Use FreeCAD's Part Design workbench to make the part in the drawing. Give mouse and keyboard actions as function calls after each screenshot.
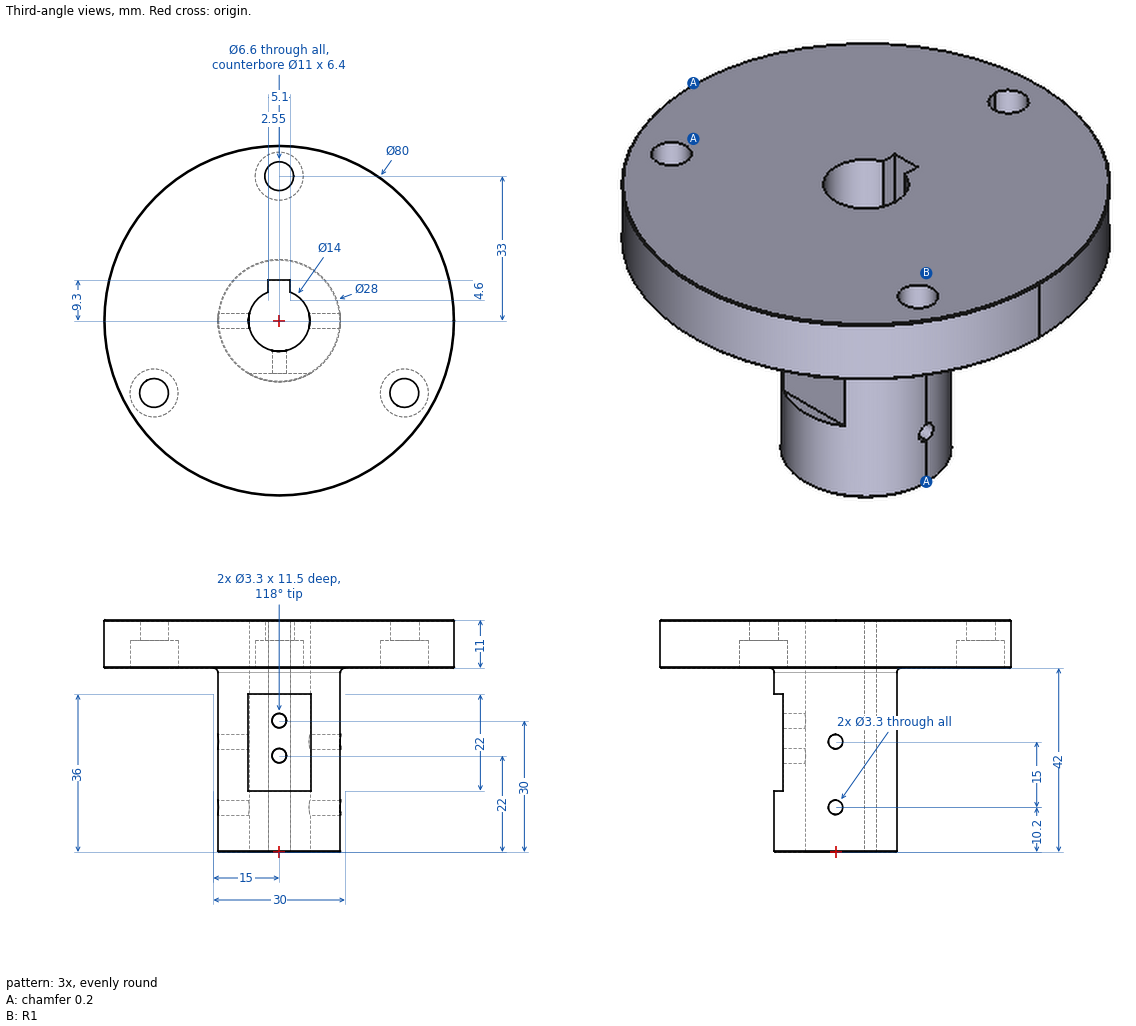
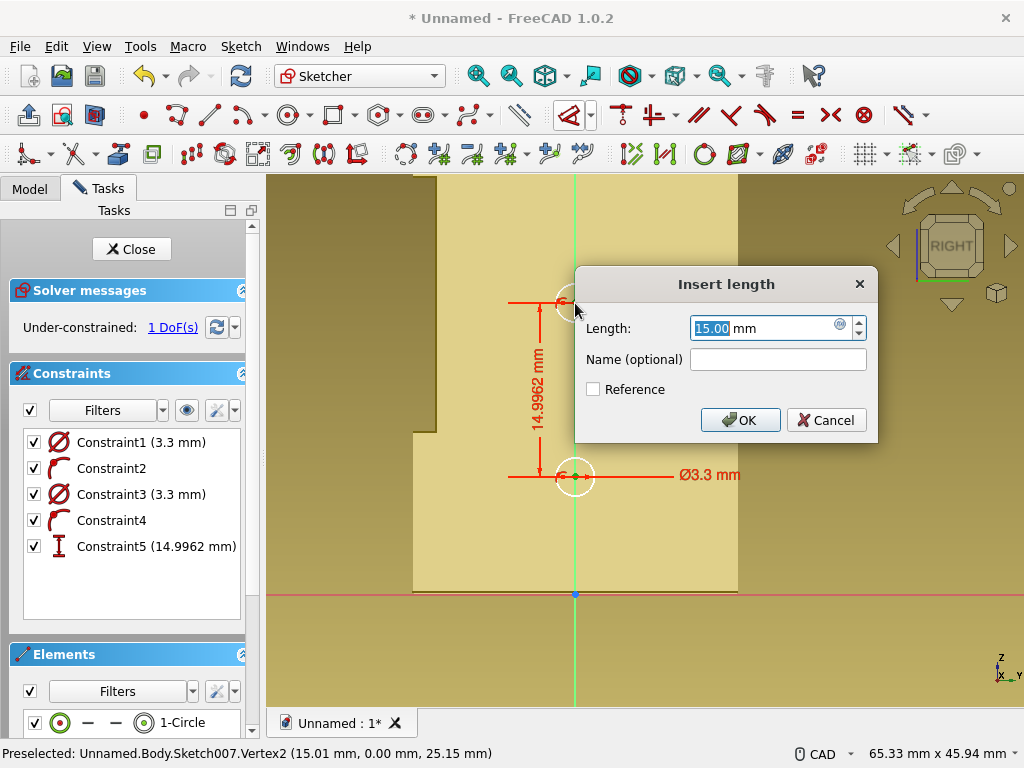
text(15)
key(Return)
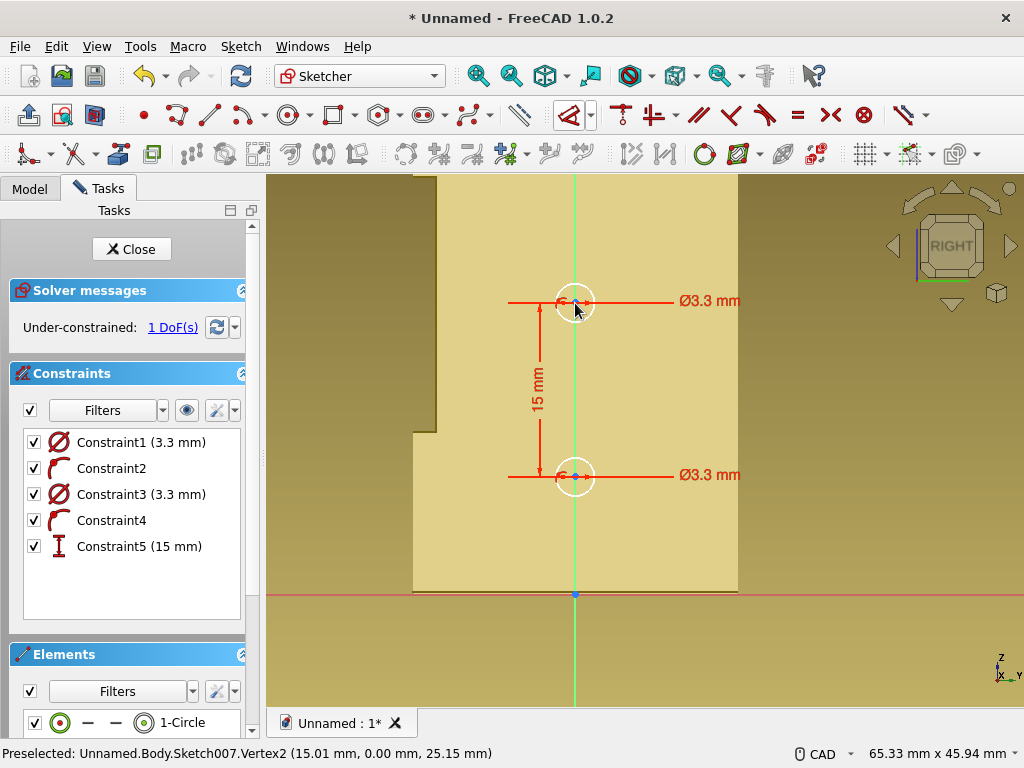
click(575, 477)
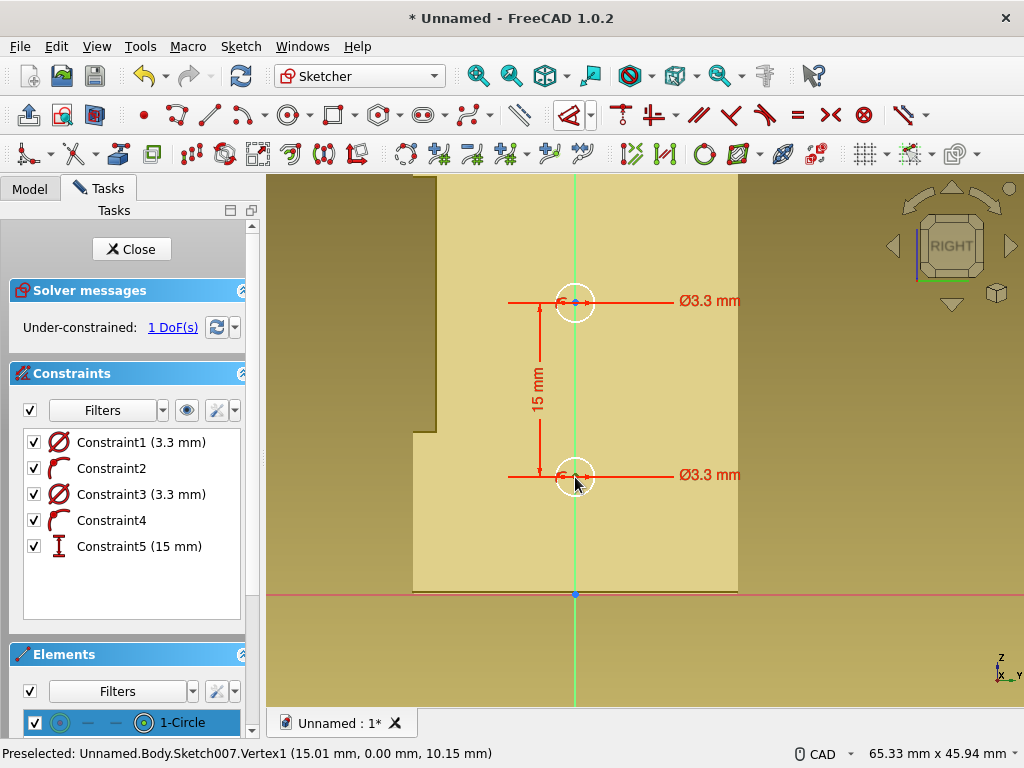
key(i)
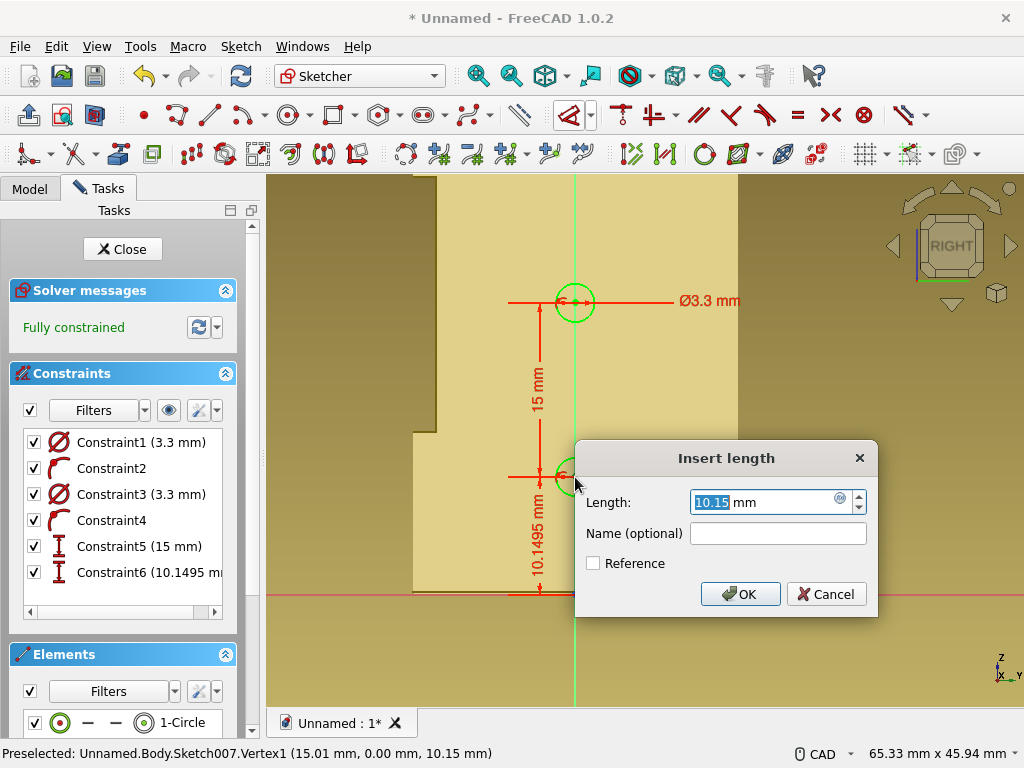
text(10.2)
key(Return)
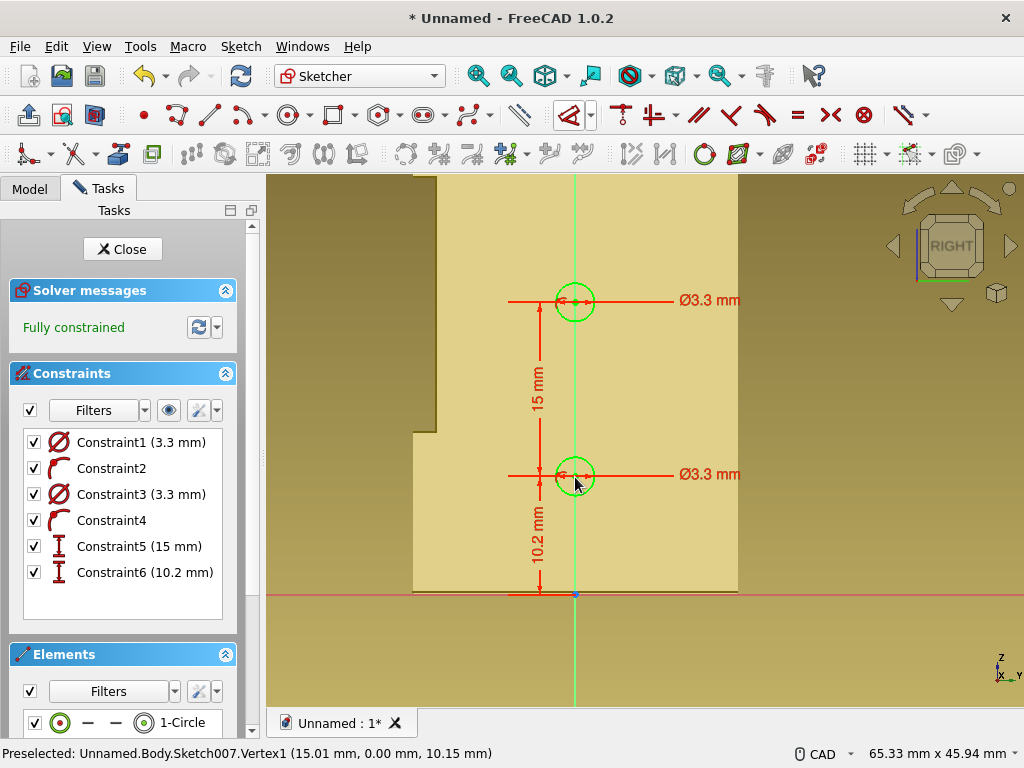
click(123, 249)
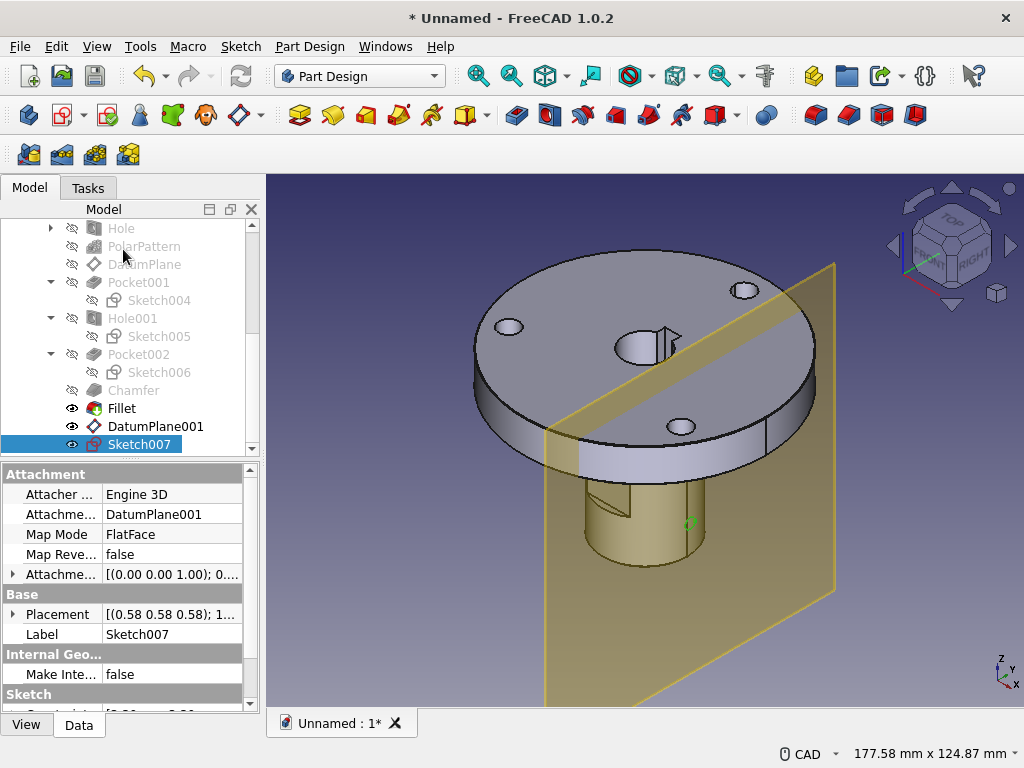
click(550, 116)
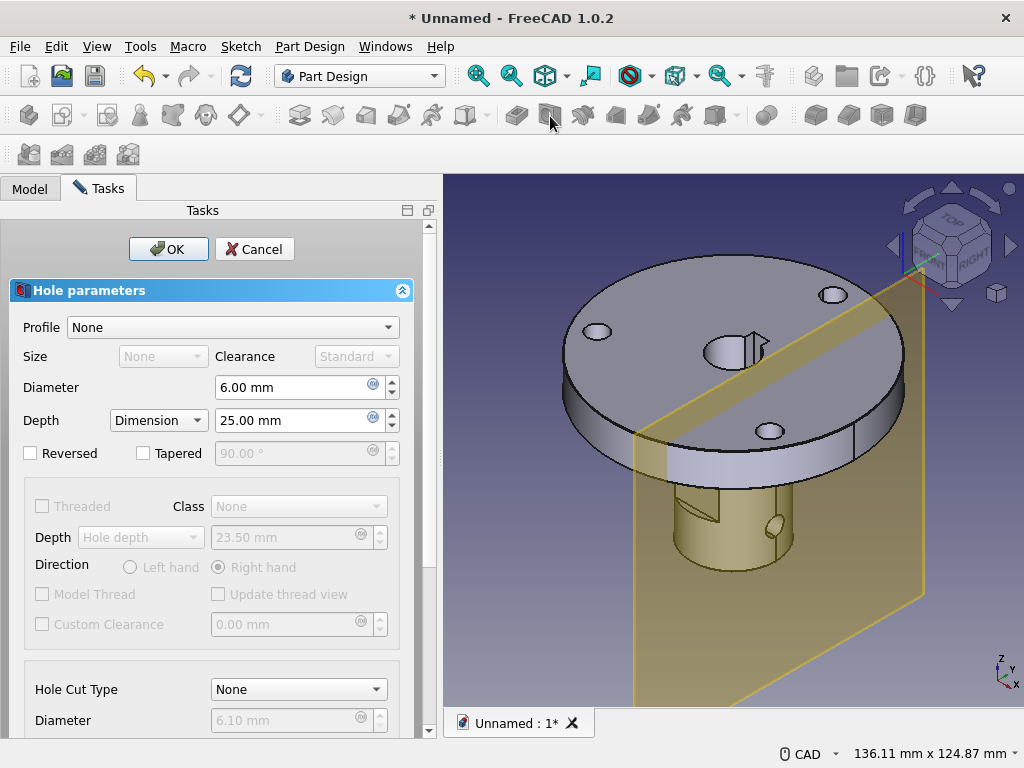
triple_click(300, 388)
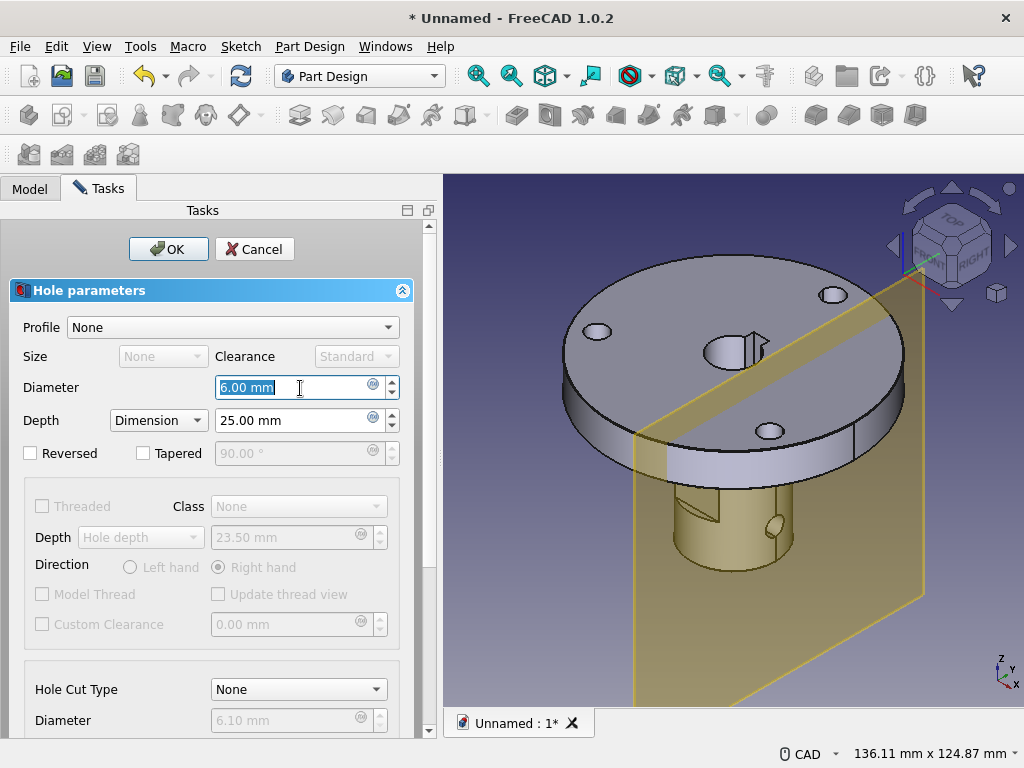
text(3.3)
key(Tab)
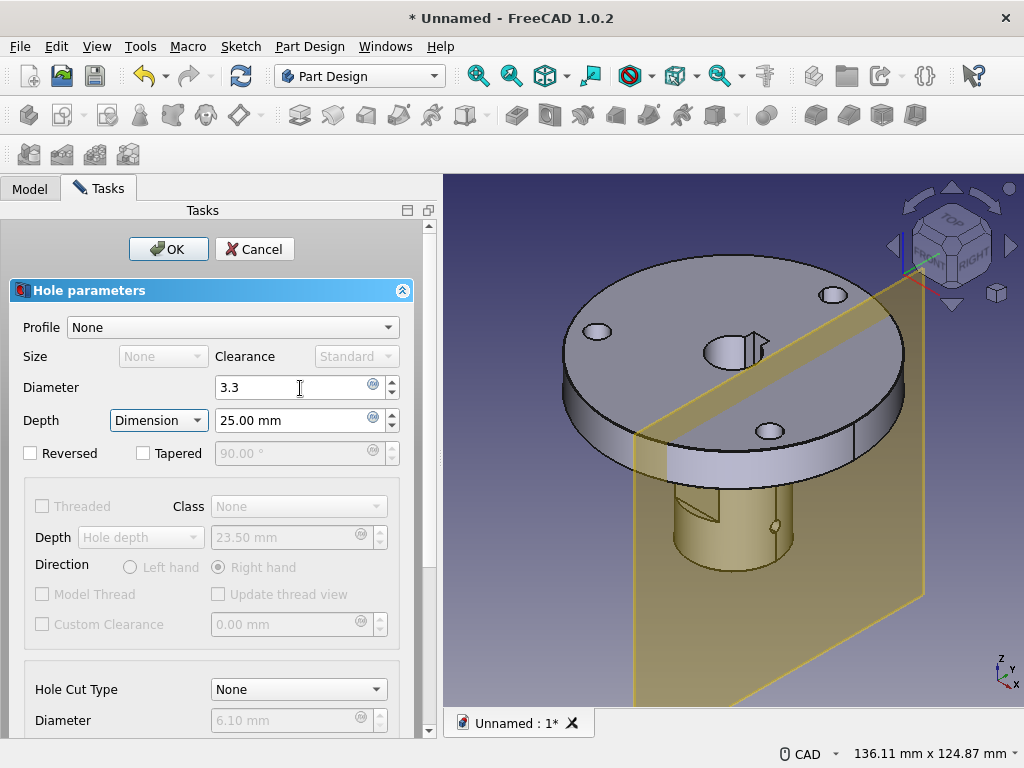
click(160, 420)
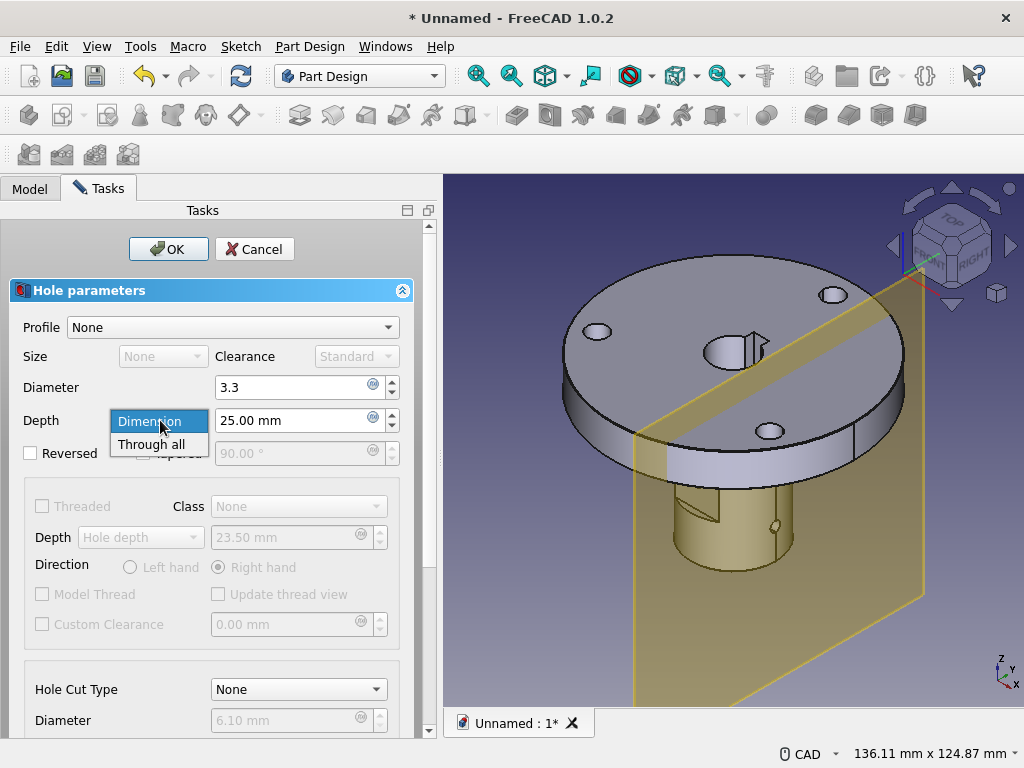
click(158, 444)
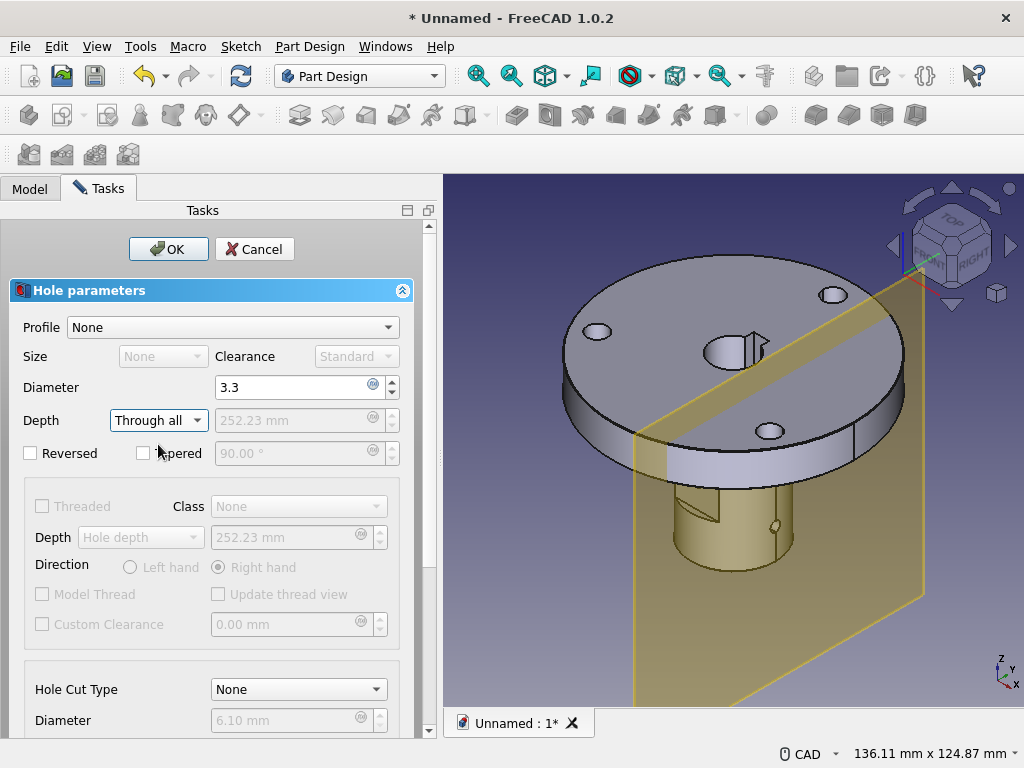
click(169, 249)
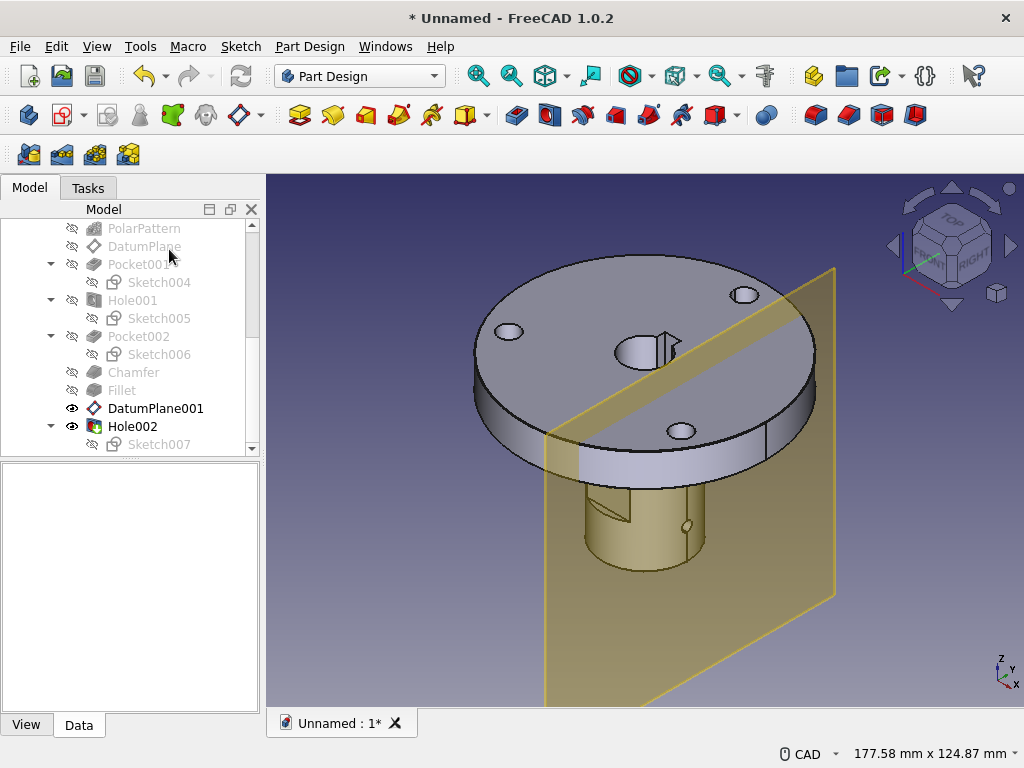
click(117, 408)
key(space)